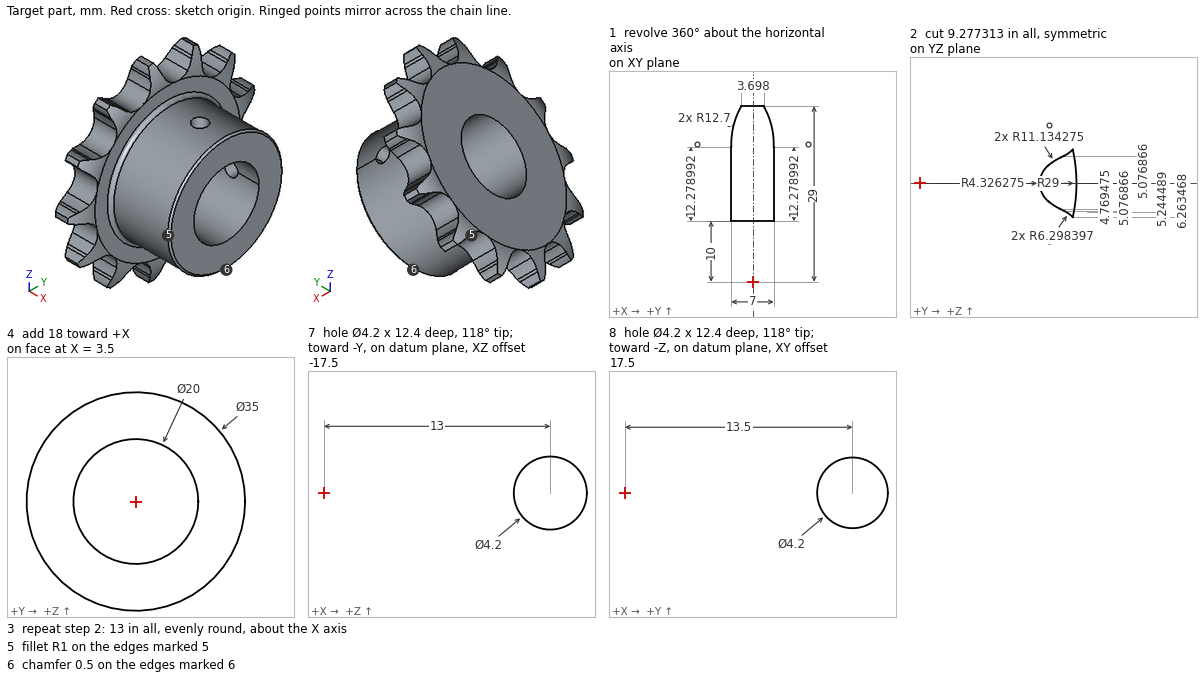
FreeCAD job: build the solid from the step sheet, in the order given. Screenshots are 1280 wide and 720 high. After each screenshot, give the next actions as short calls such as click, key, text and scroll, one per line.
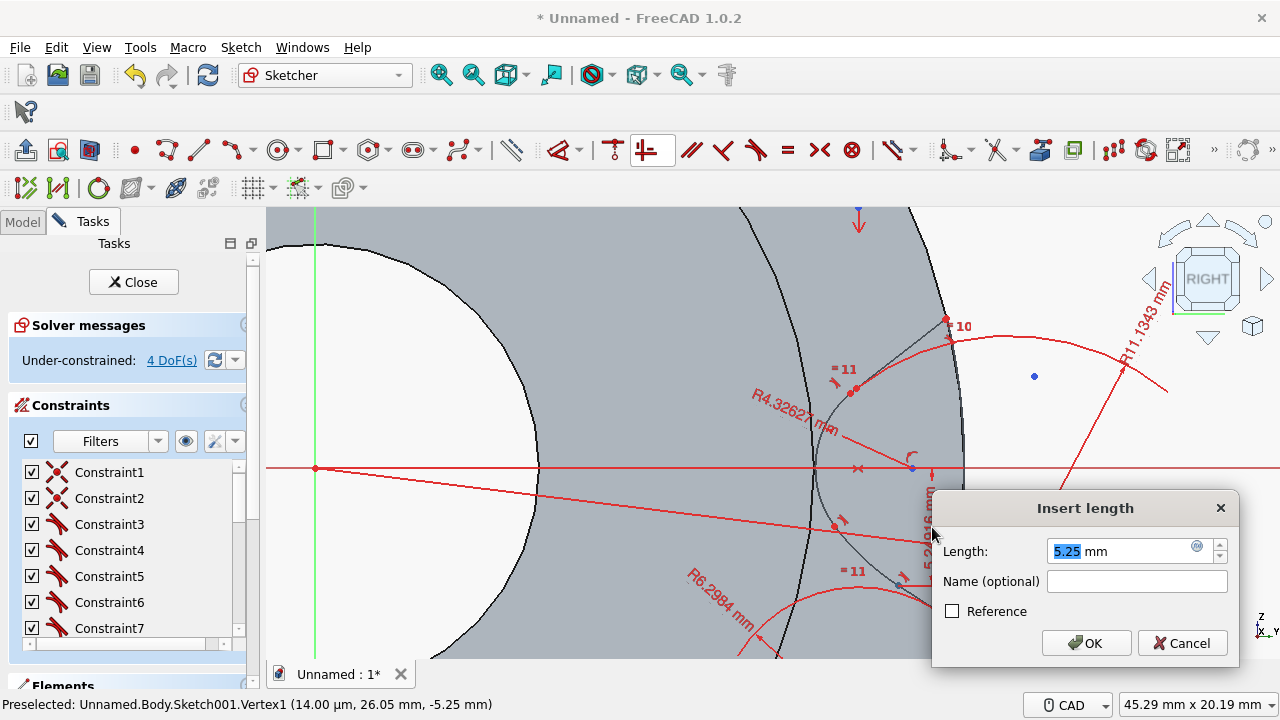
text(4.769475)
key(Return)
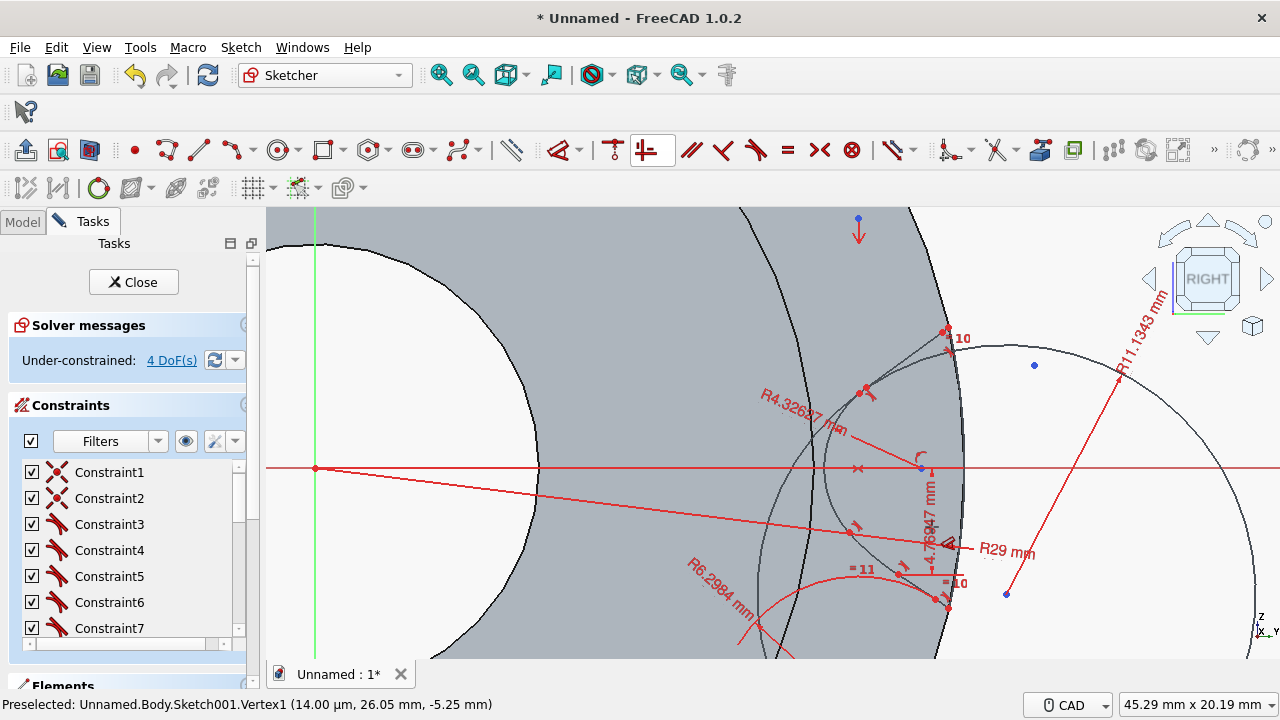
click(936, 599)
click(970, 580)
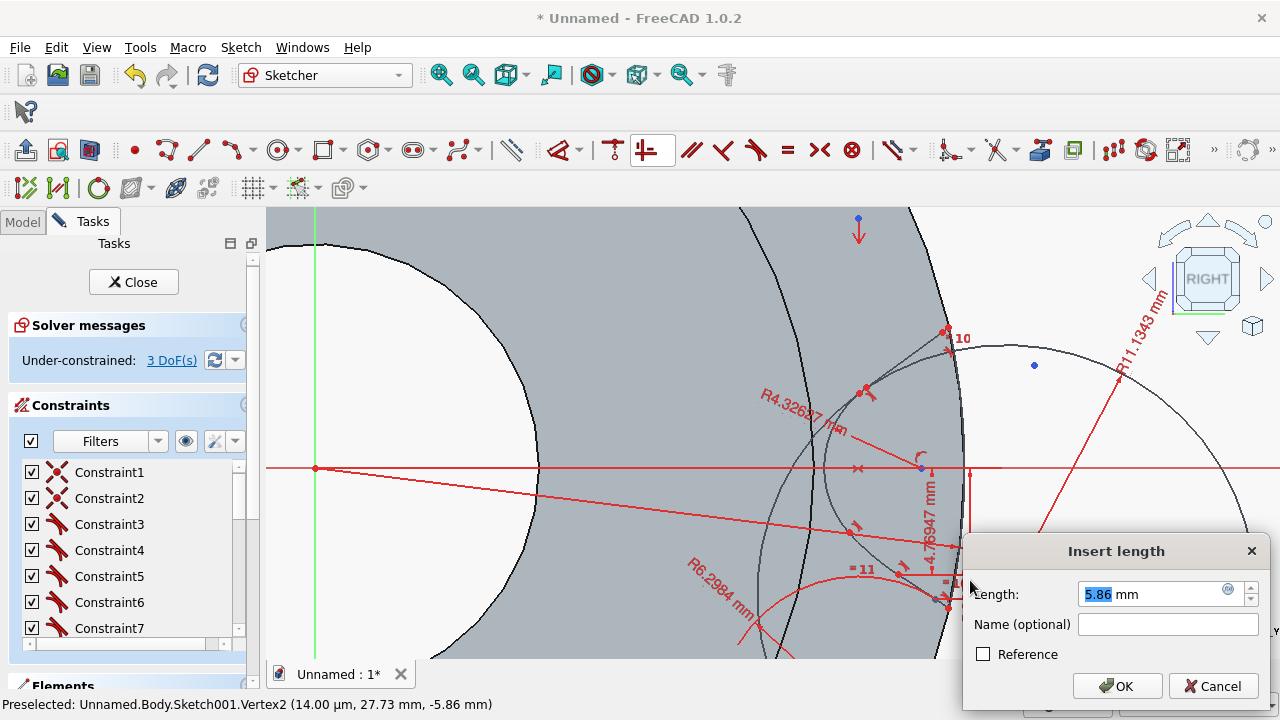
text(5.076866)
key(Return)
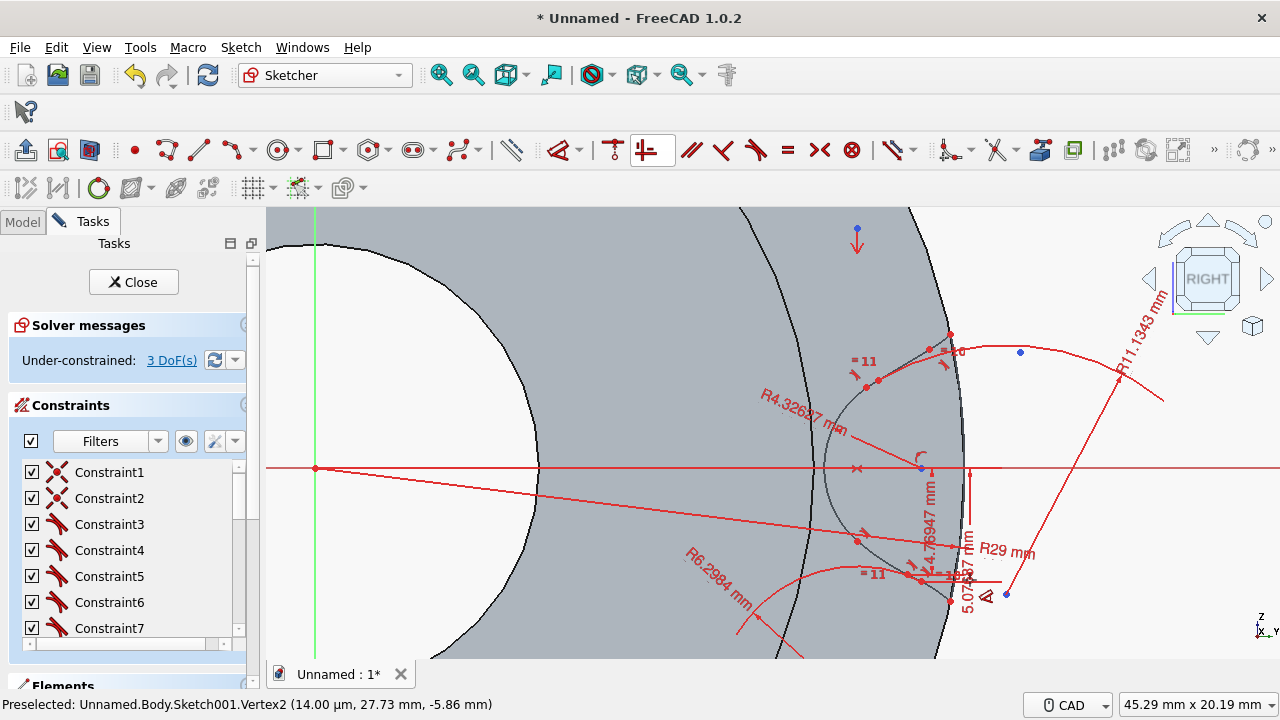
click(930, 350)
click(988, 409)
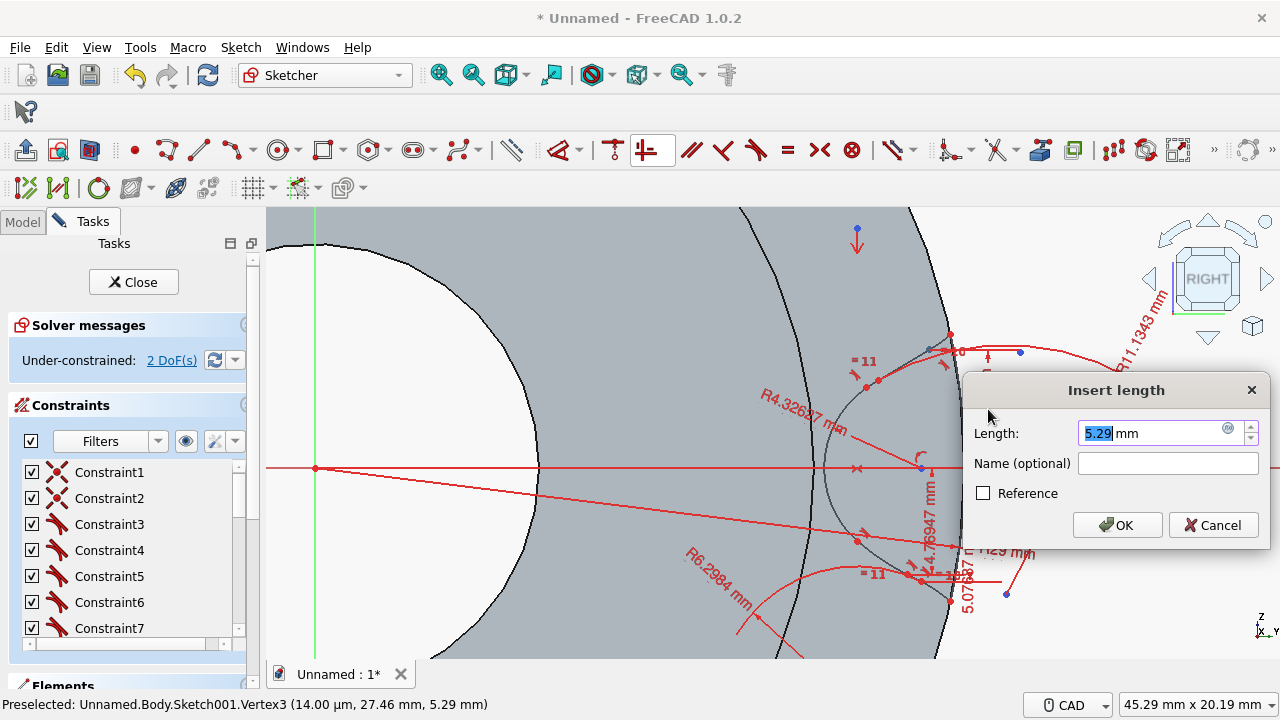
text(5.076866)
key(Return)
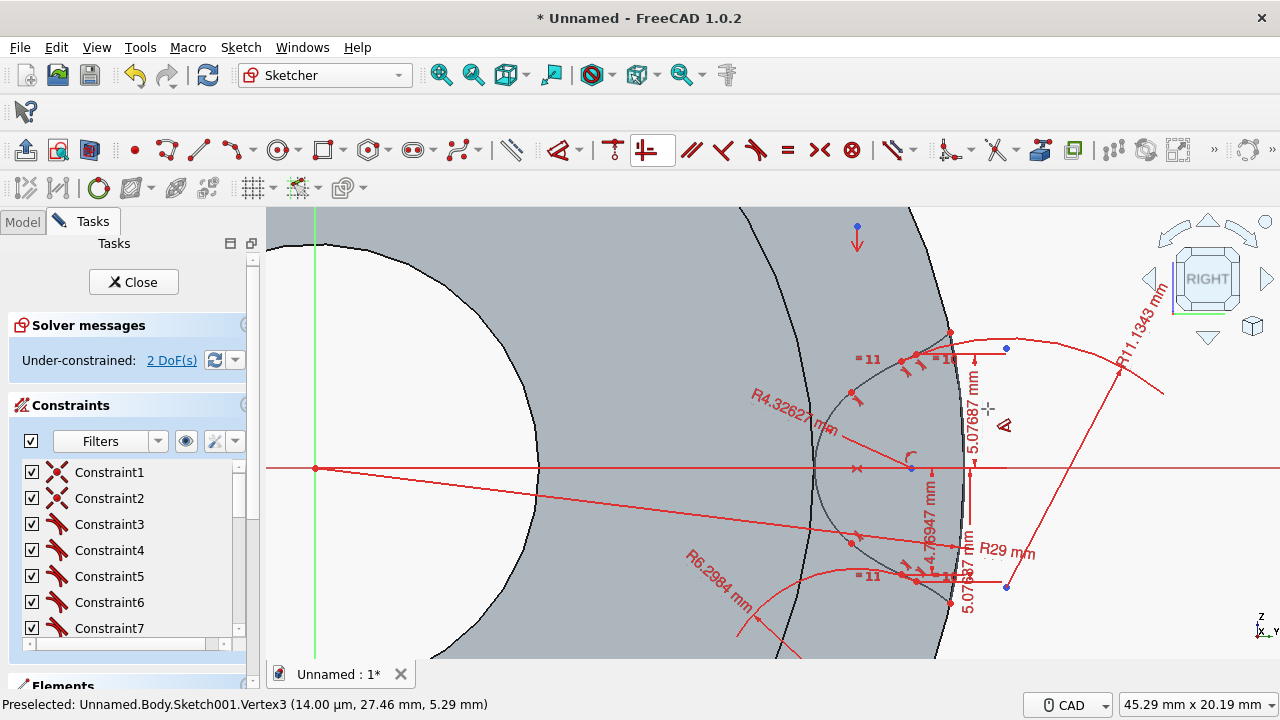
click(950, 603)
click(984, 505)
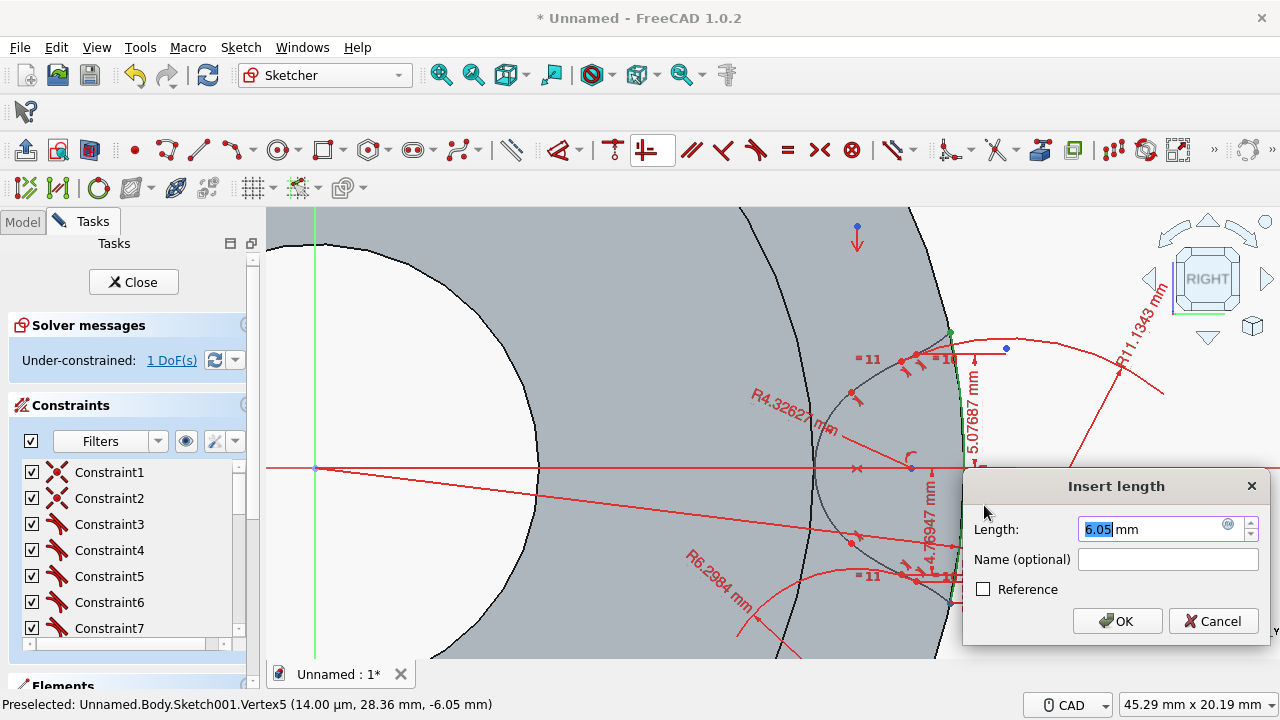
text(6.263468)
key(Return)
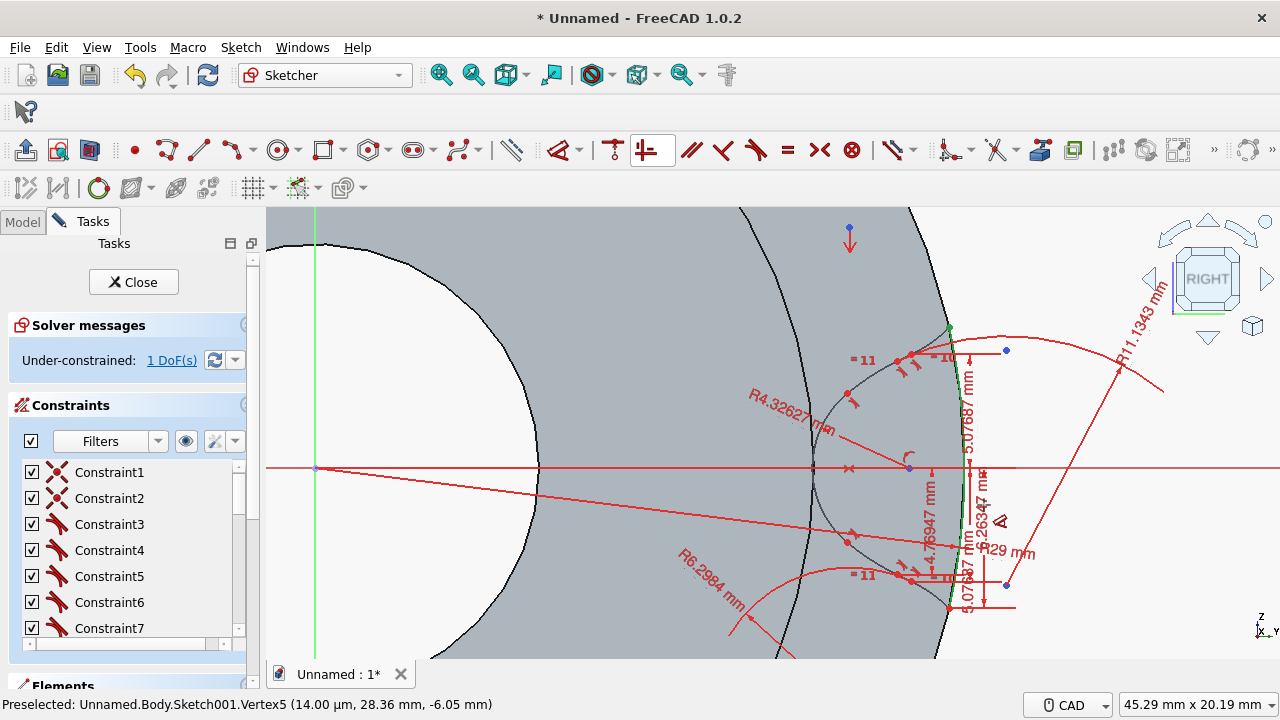
click(1006, 585)
click(1040, 527)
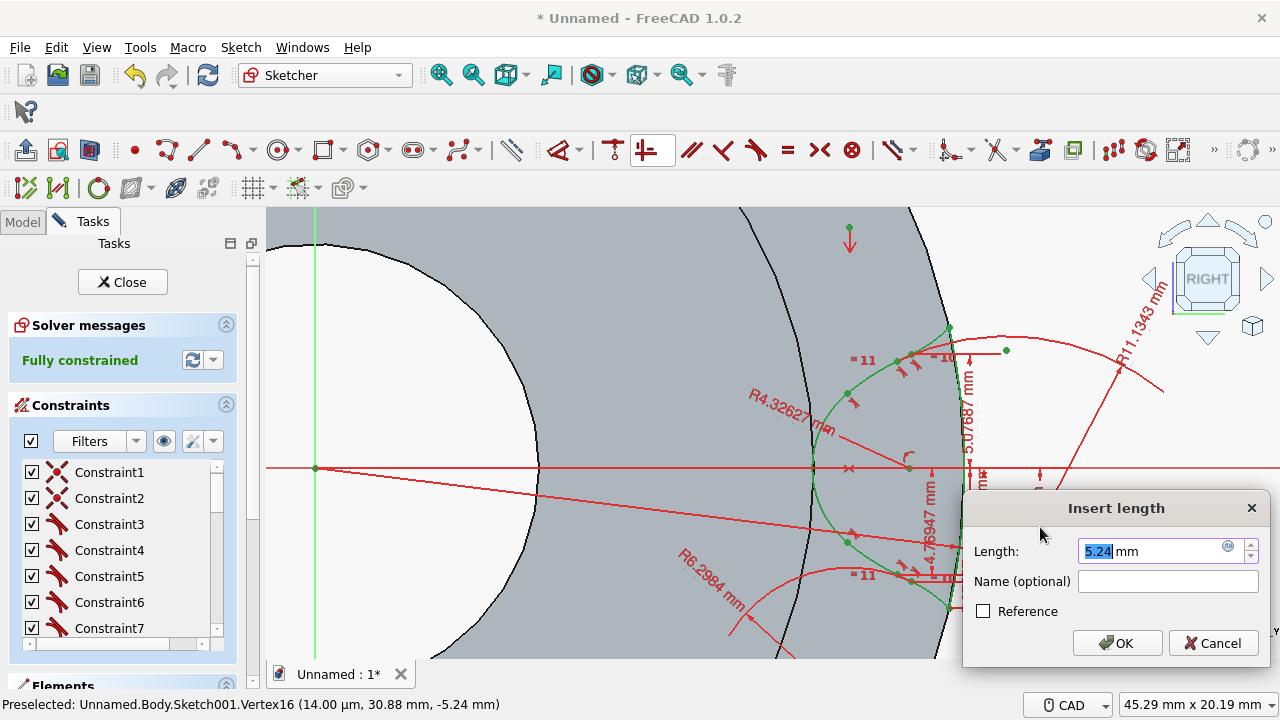
text(5.244489)
key(Return)
key(Escape)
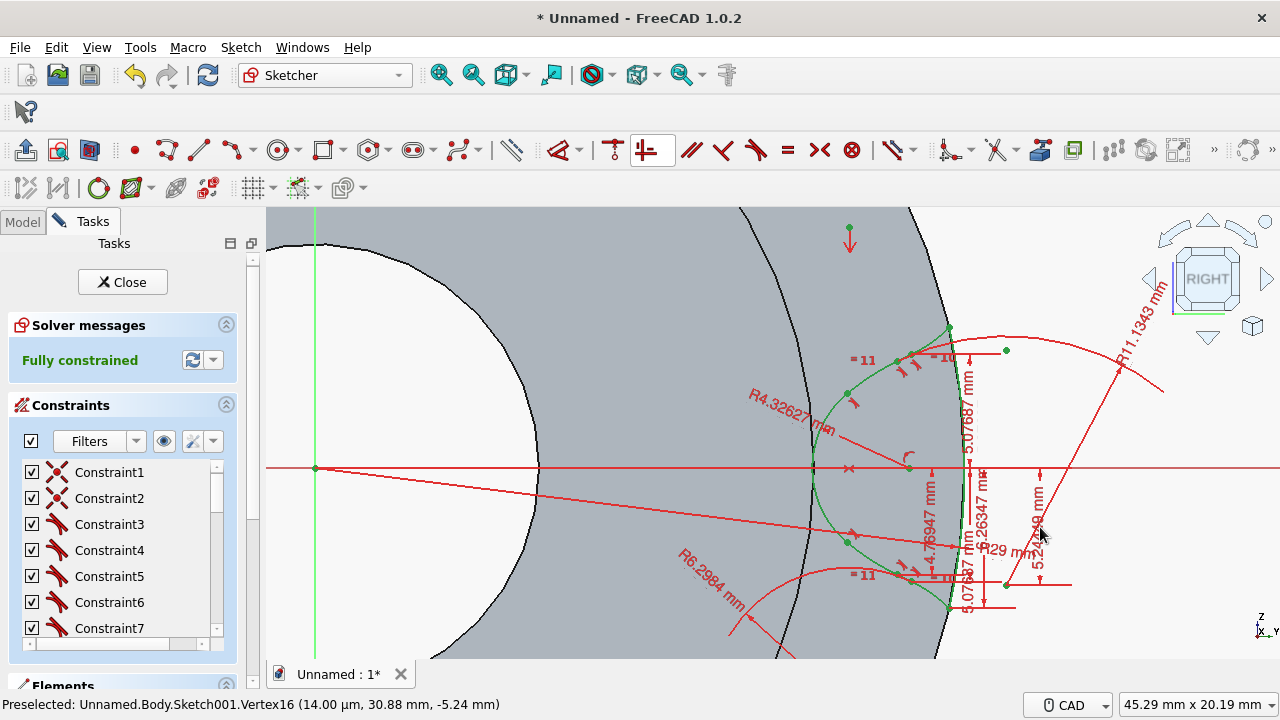
click(123, 282)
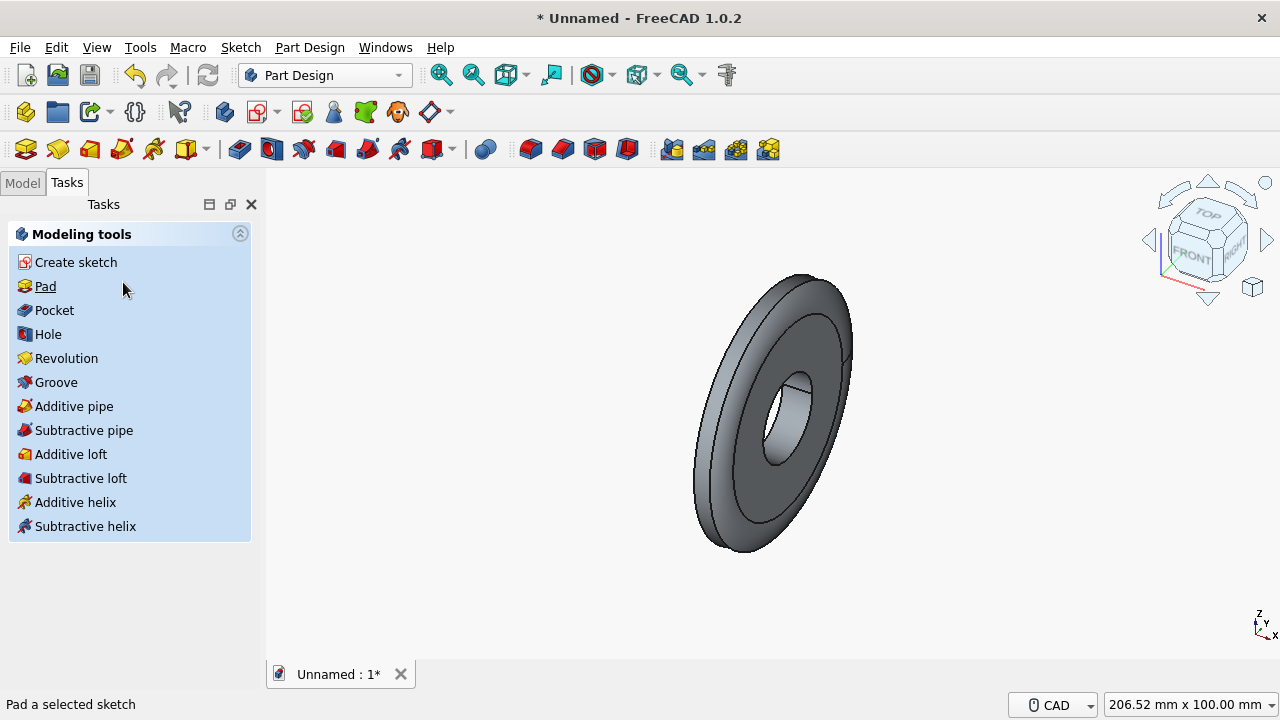
click(240, 150)